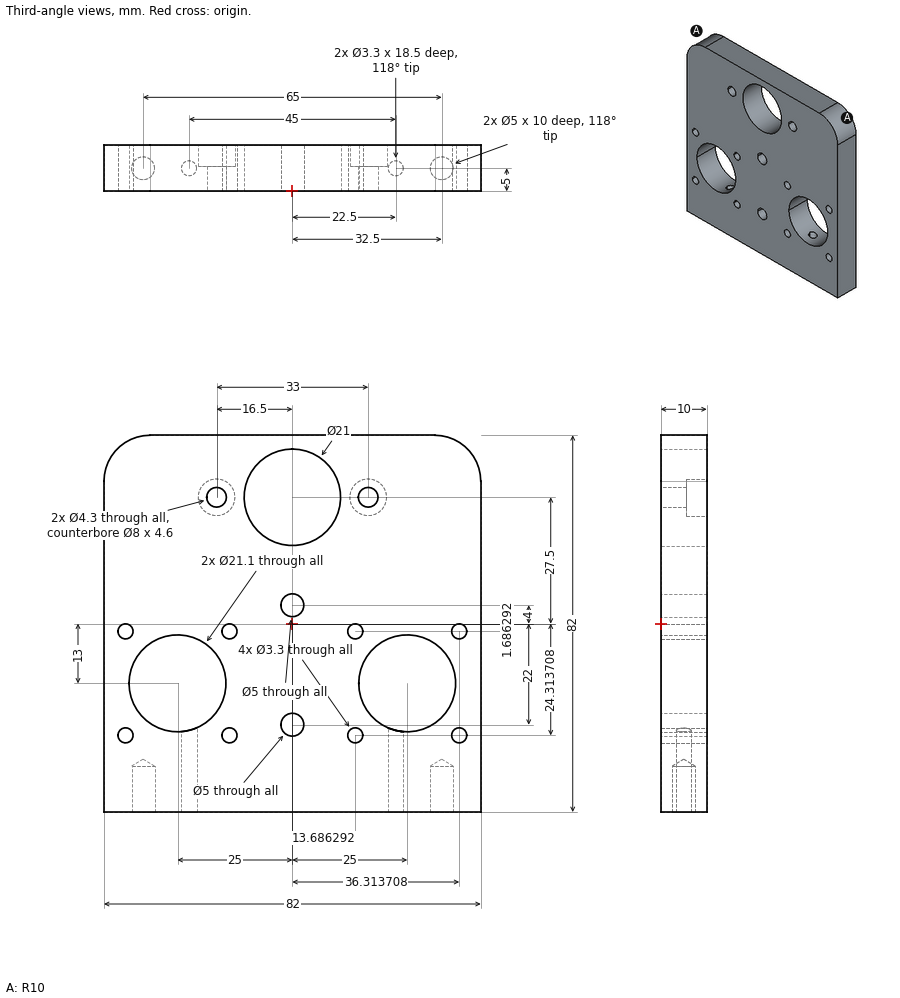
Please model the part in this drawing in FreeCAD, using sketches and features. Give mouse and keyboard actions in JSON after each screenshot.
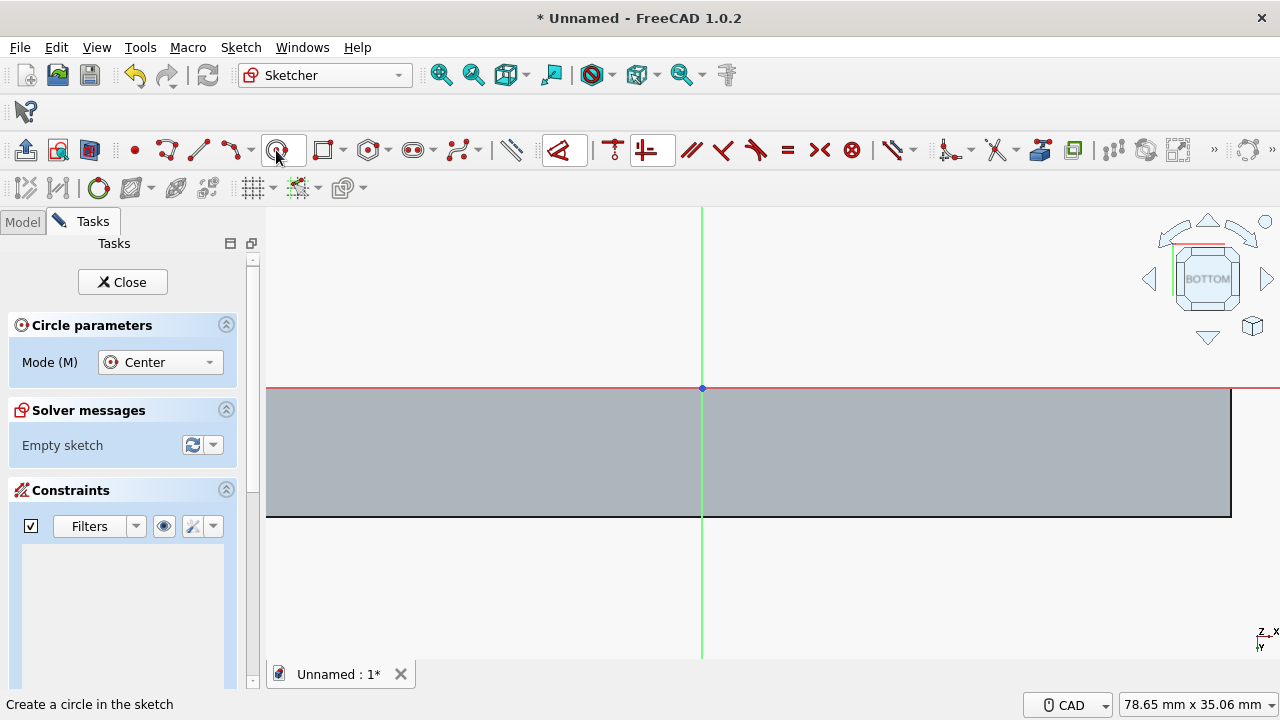
{"action": "left_click", "coordinate": [992, 453]}
{"action": "left_click", "coordinate": [1007, 438]}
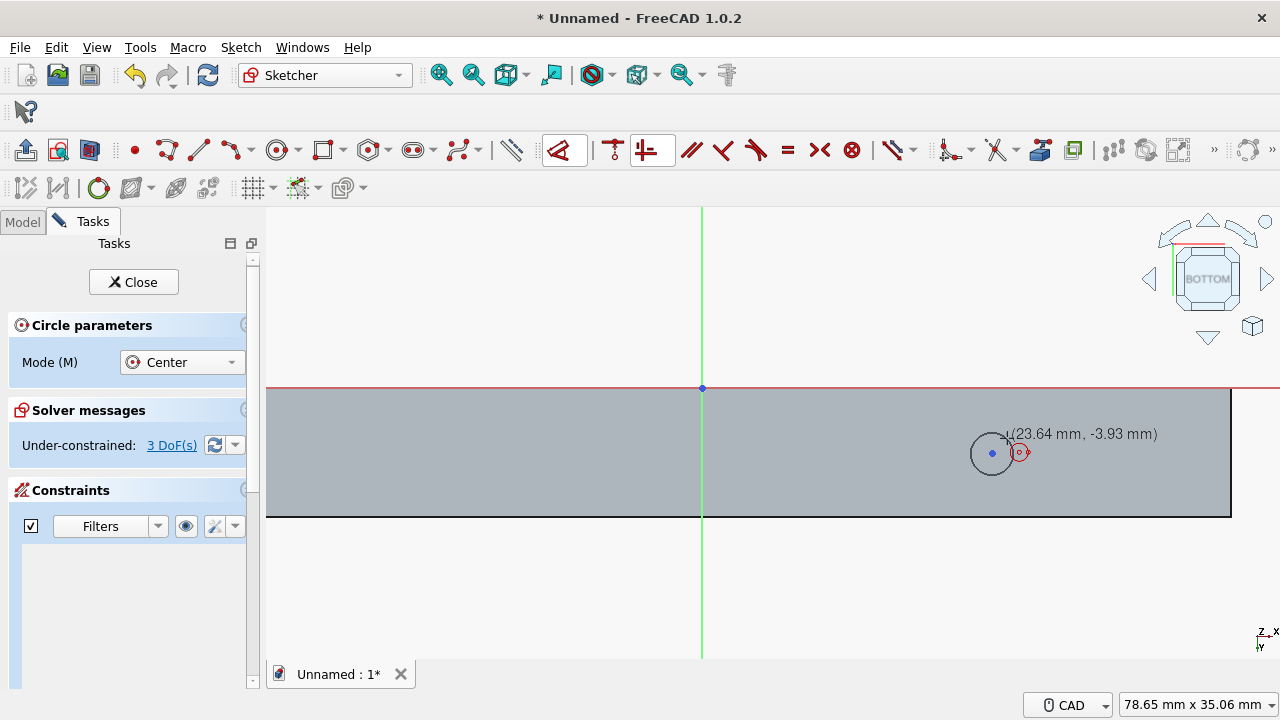
{"action": "left_click", "coordinate": [412, 453]}
{"action": "left_click", "coordinate": [427, 438]}
{"action": "key", "text": "Escape"}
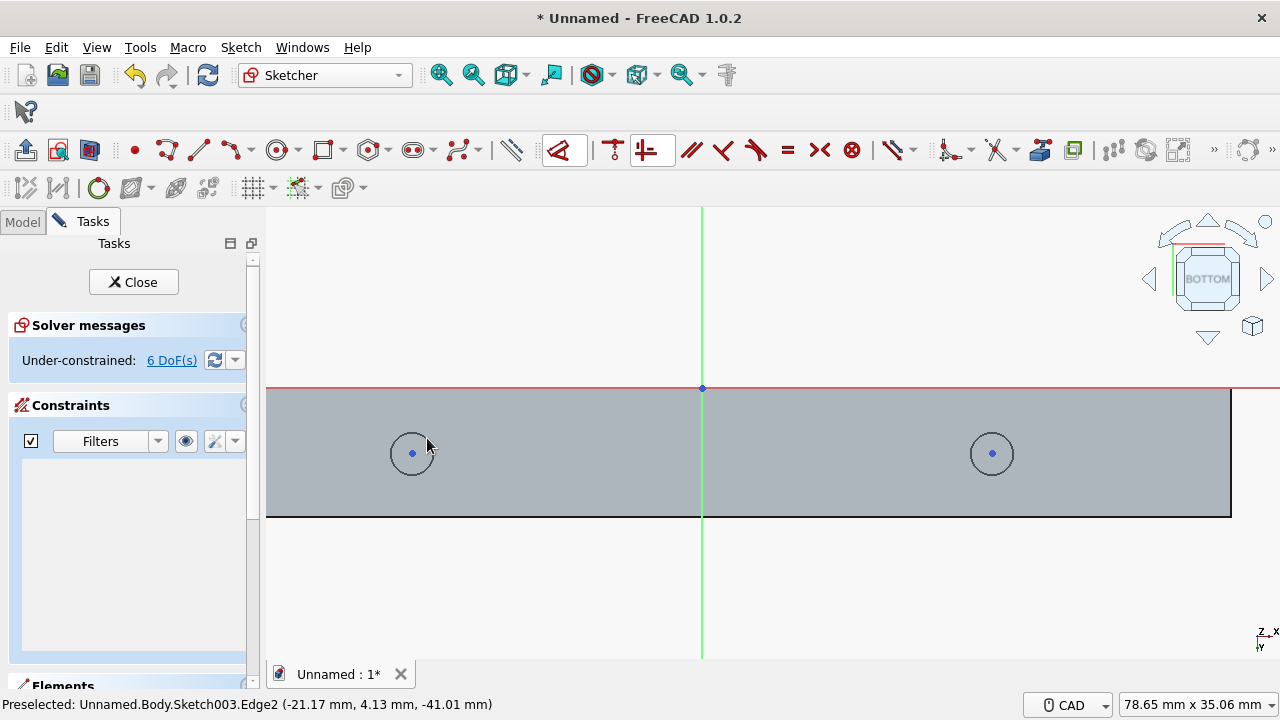
{"action": "left_click", "coordinate": [1007, 439]}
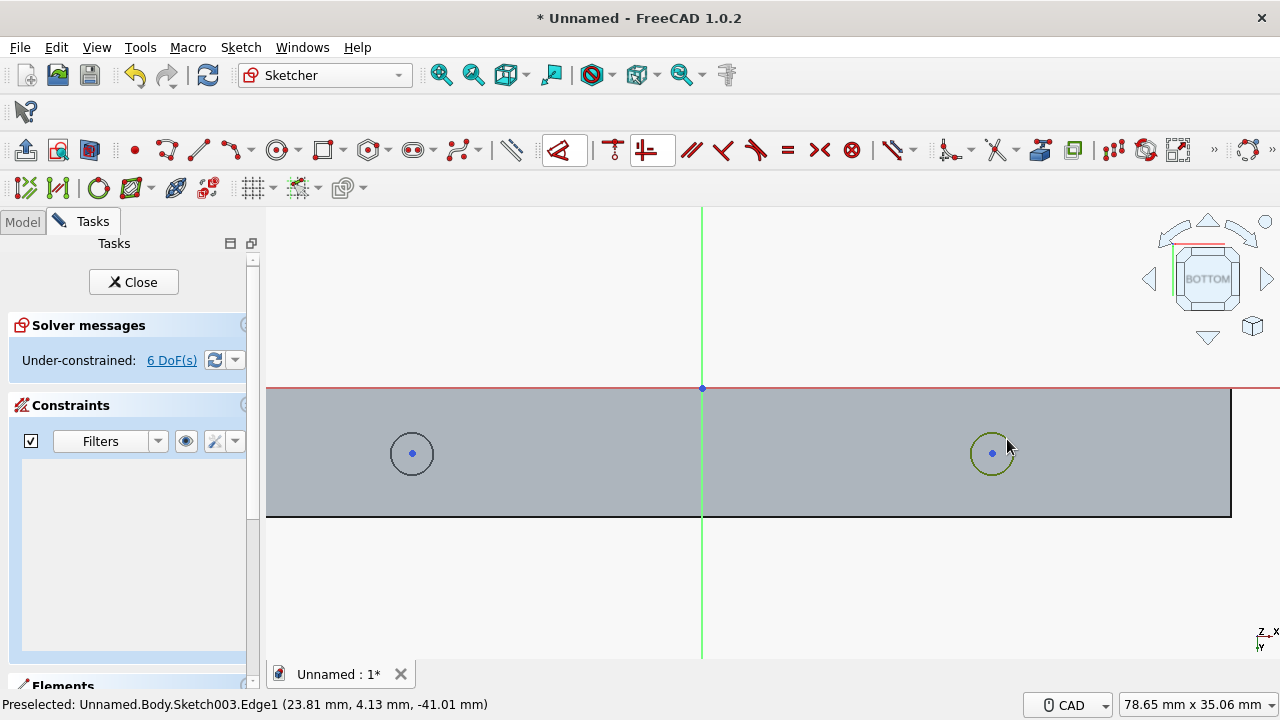
{"action": "left_click", "coordinate": [427, 439]}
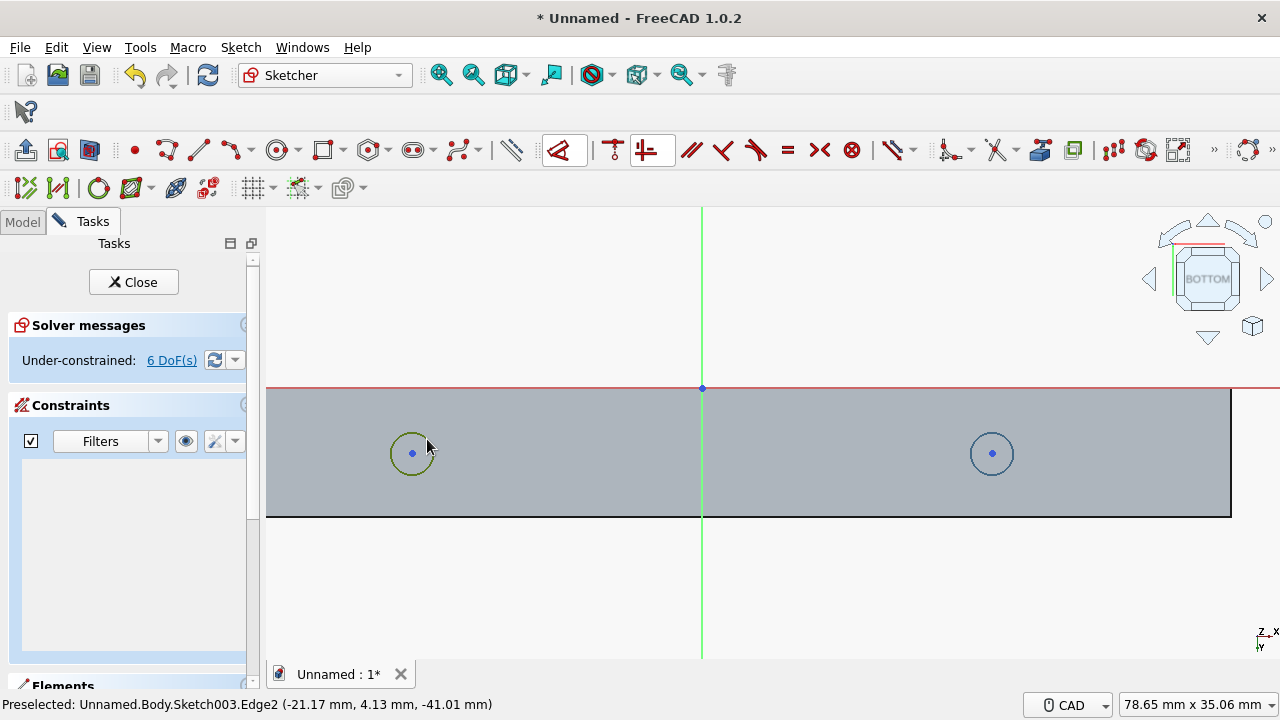
{"action": "left_click", "coordinate": [788, 150]}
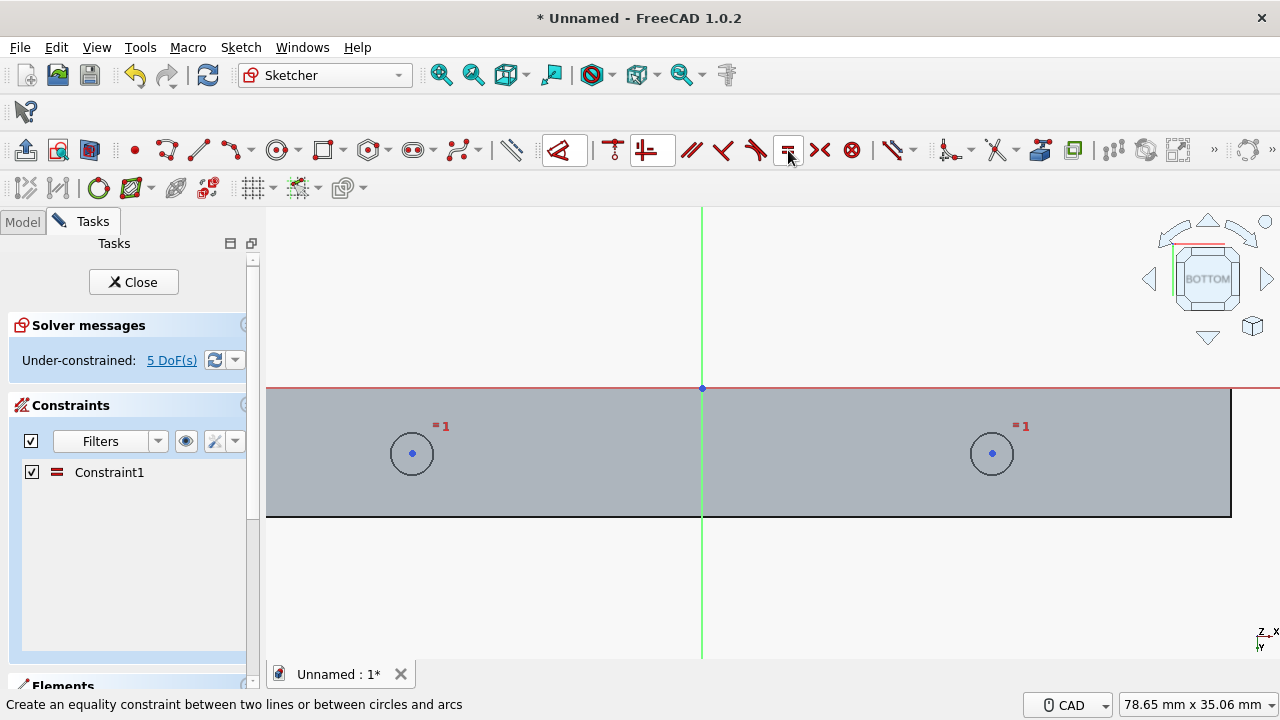
{"action": "left_click", "coordinate": [1007, 439]}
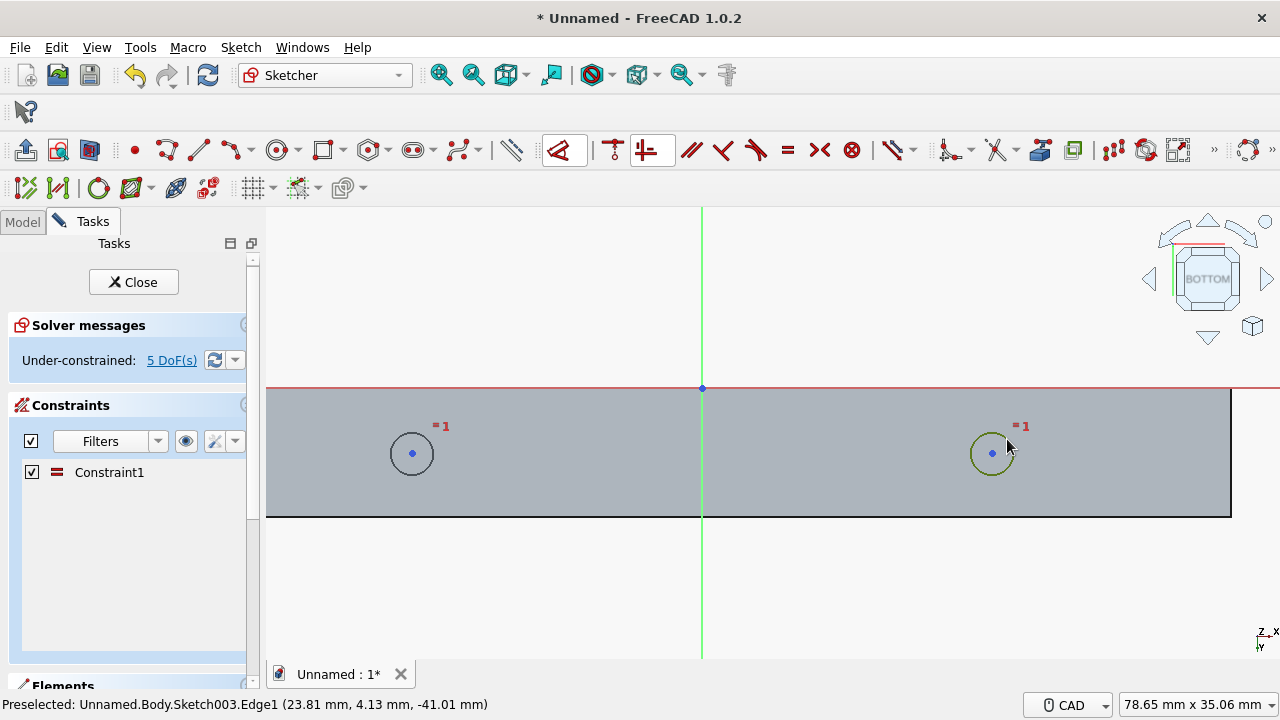
{"action": "key", "text": "k o"}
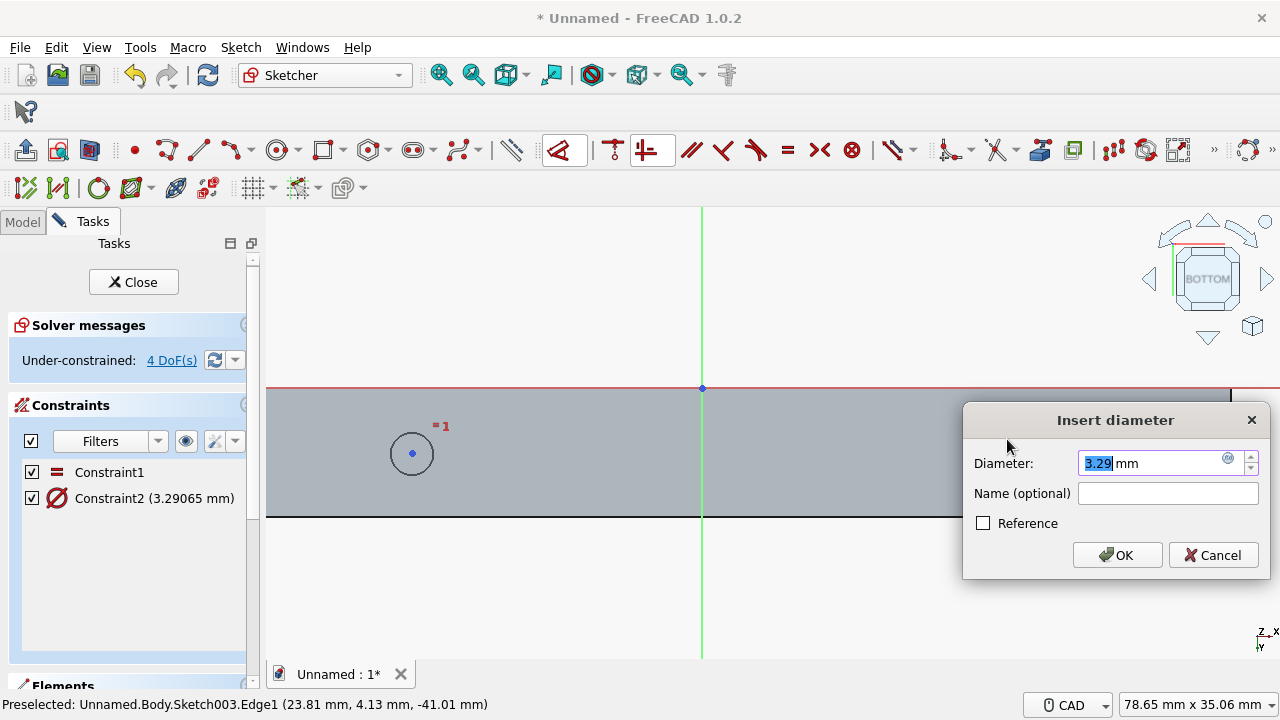
{"action": "type", "text": "3.3"}
{"action": "key", "text": "Return"}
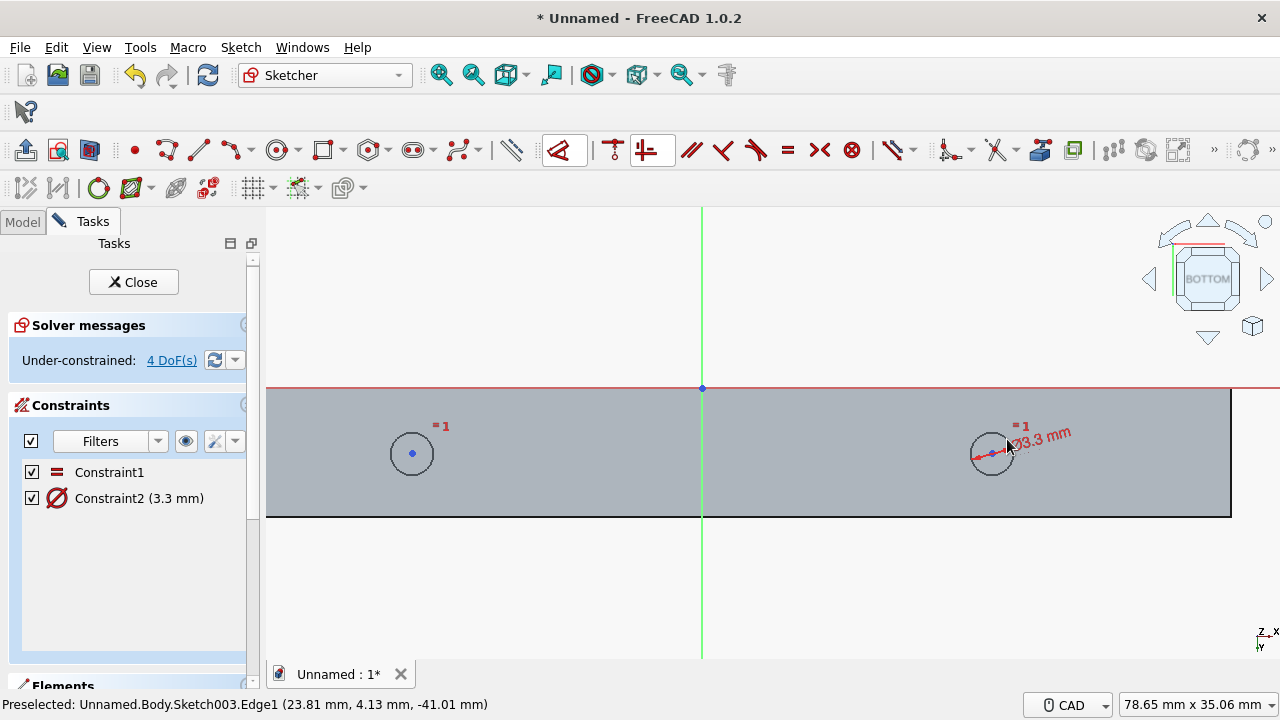
{"action": "left_click", "coordinate": [992, 454]}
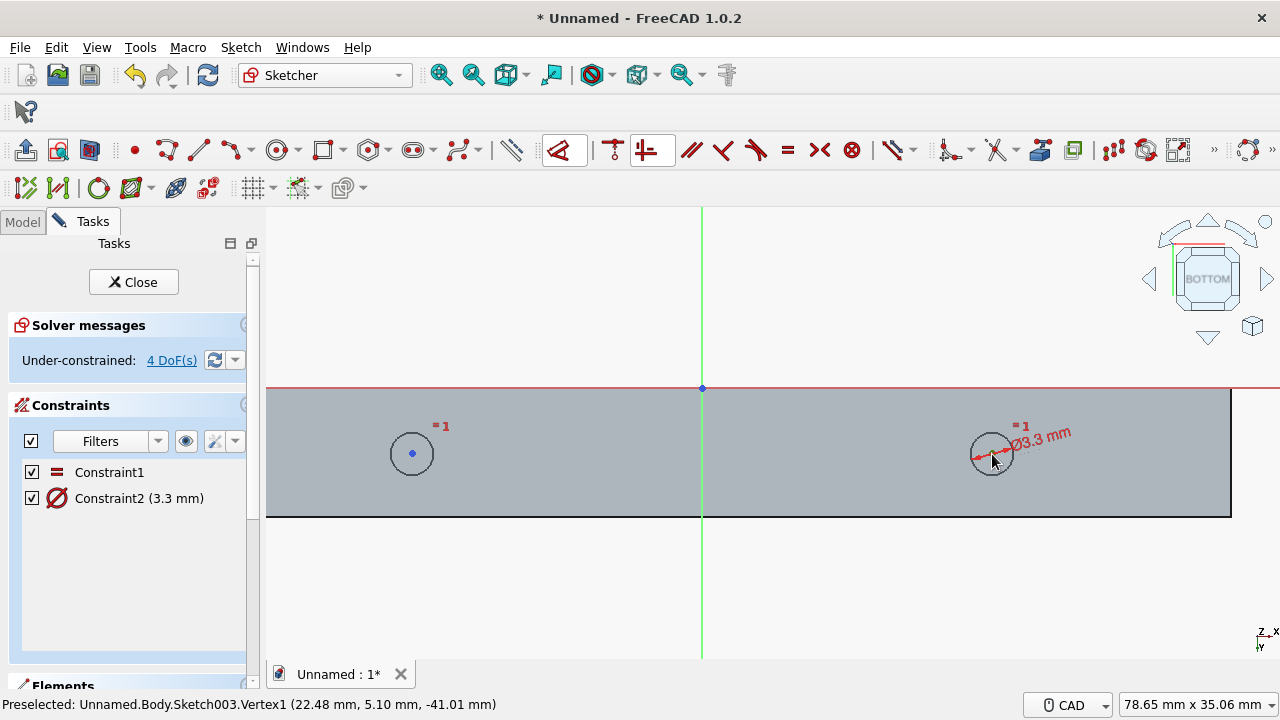
{"action": "left_click", "coordinate": [582, 150]}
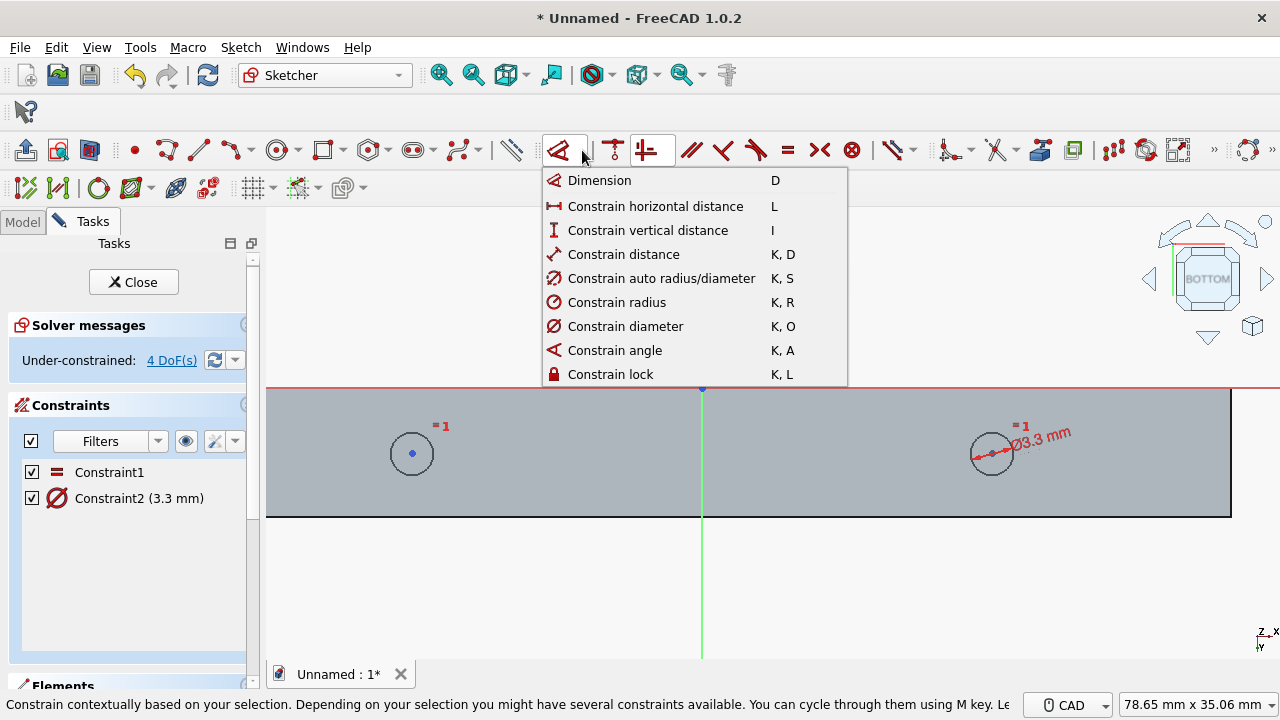
{"action": "left_click", "coordinate": [695, 230]}